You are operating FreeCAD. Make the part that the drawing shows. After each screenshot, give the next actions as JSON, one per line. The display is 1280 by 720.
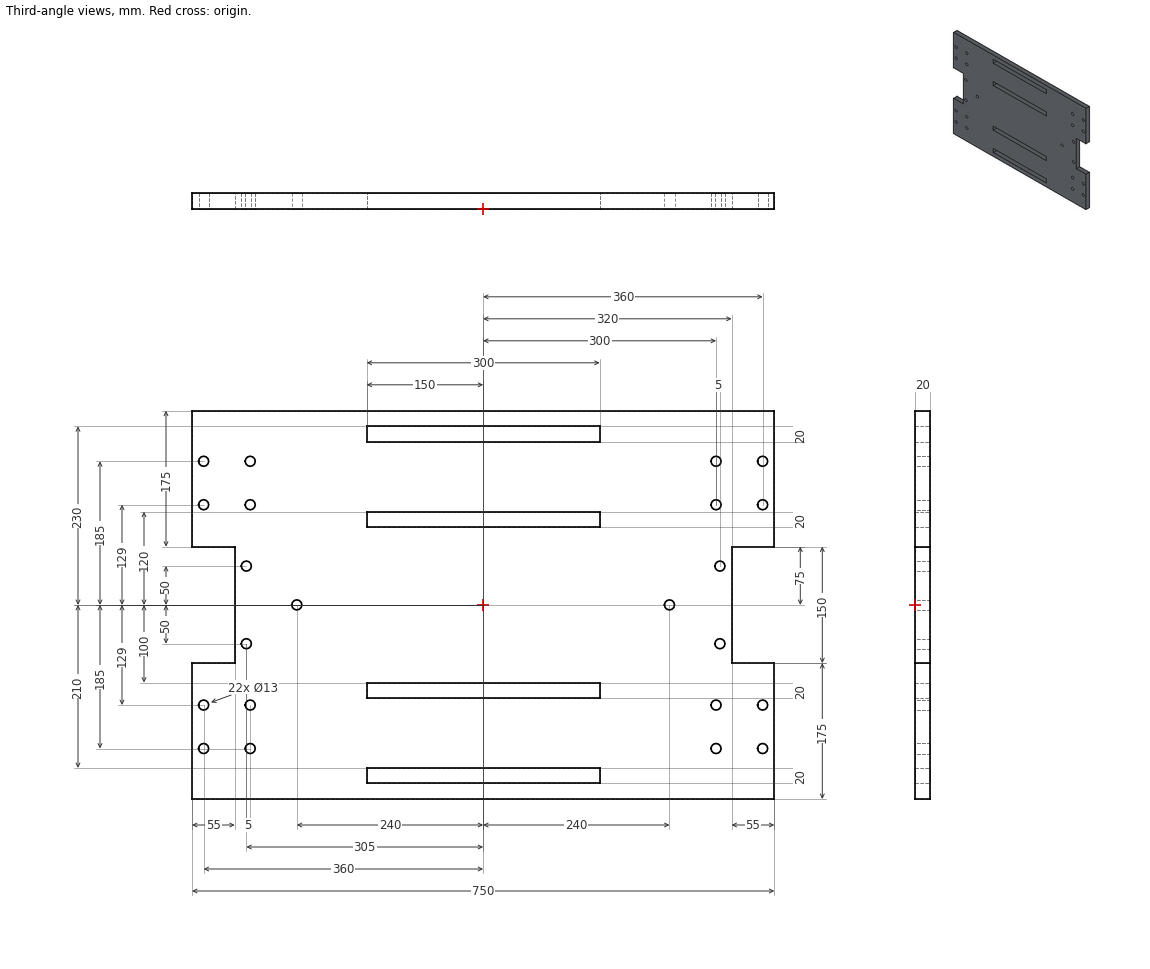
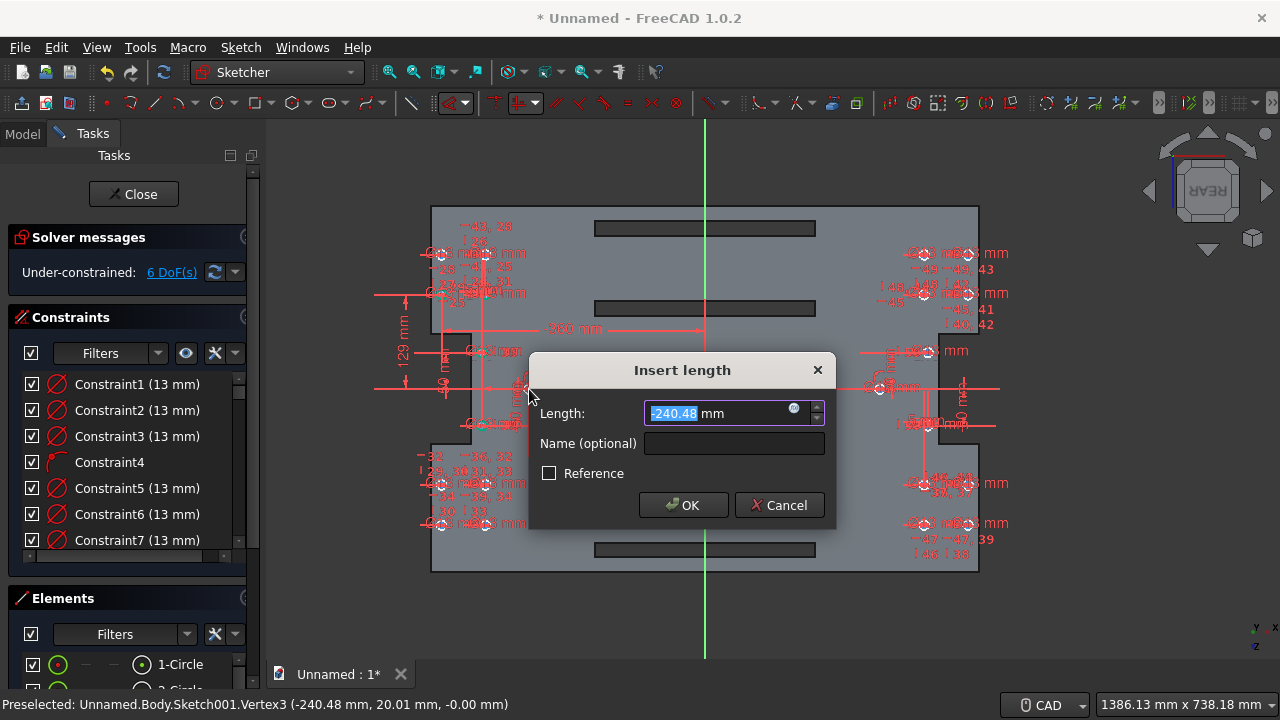
{"action": "type", "text": "-240"}
{"action": "key", "text": "Return"}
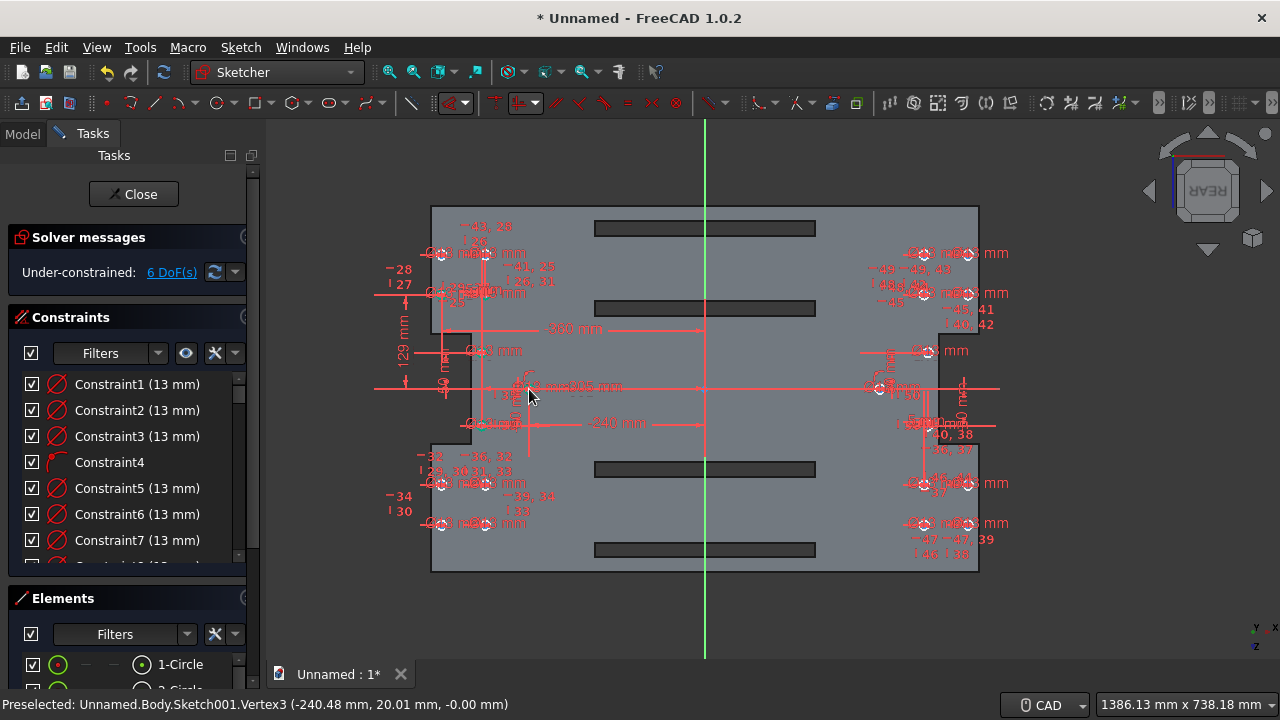
{"action": "left_click", "coordinate": [485, 255]}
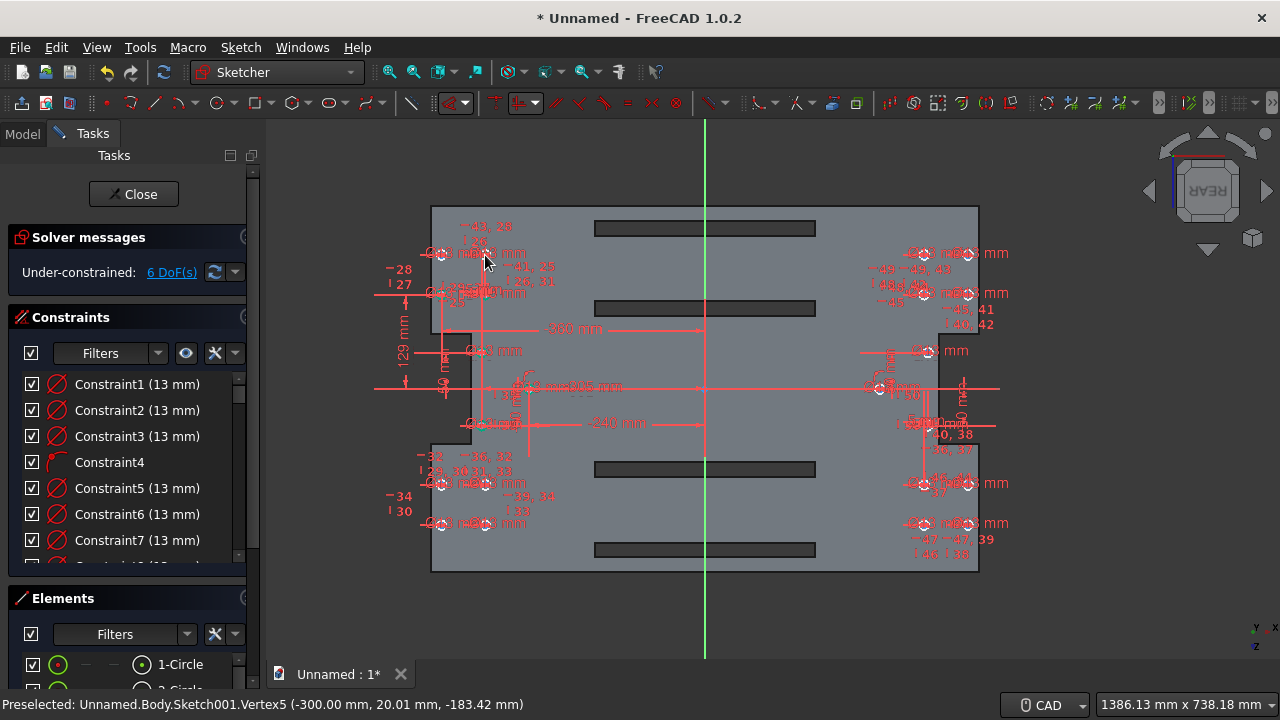
{"action": "left_click", "coordinate": [468, 104]}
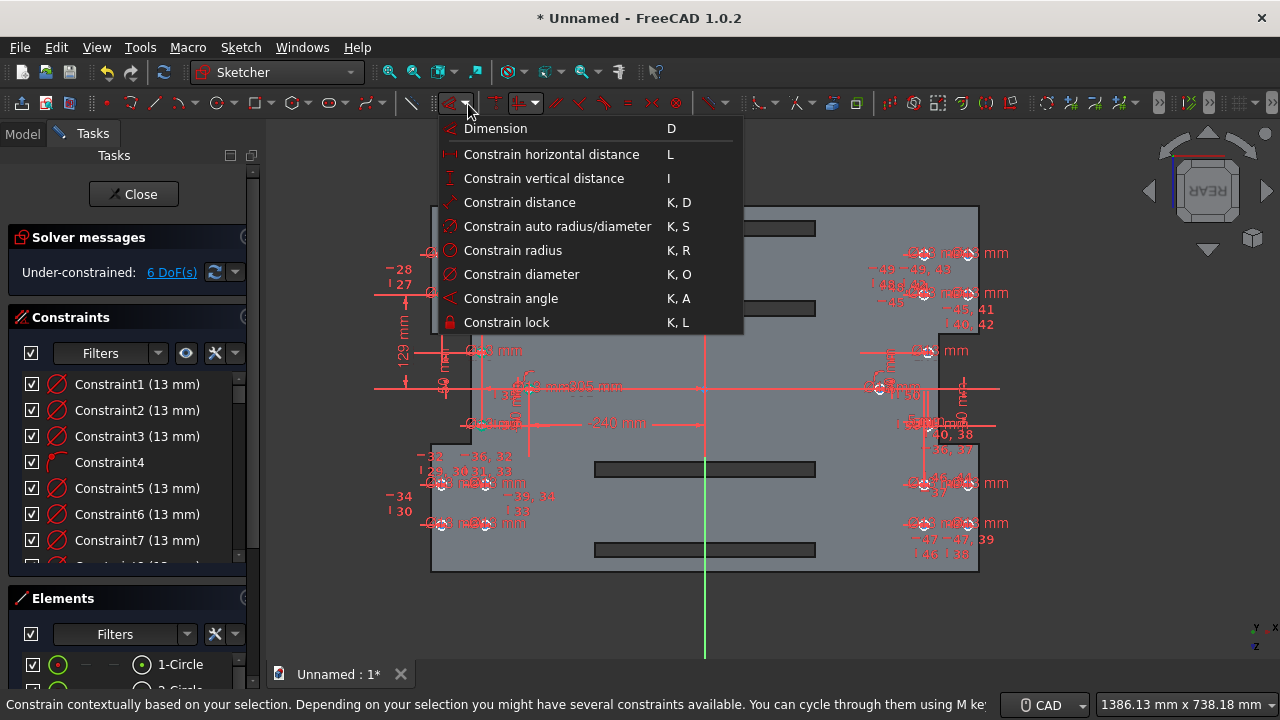
{"action": "left_click", "coordinate": [591, 178]}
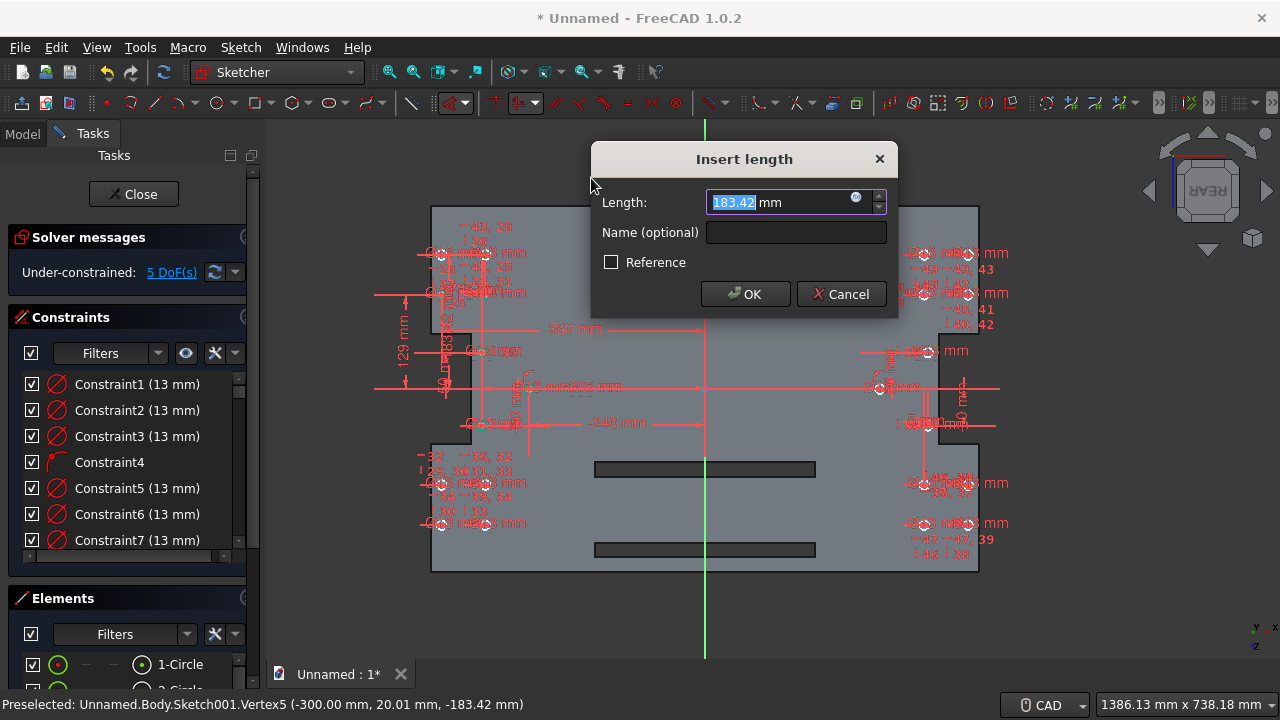
{"action": "type", "text": "185"}
{"action": "key", "text": "Return"}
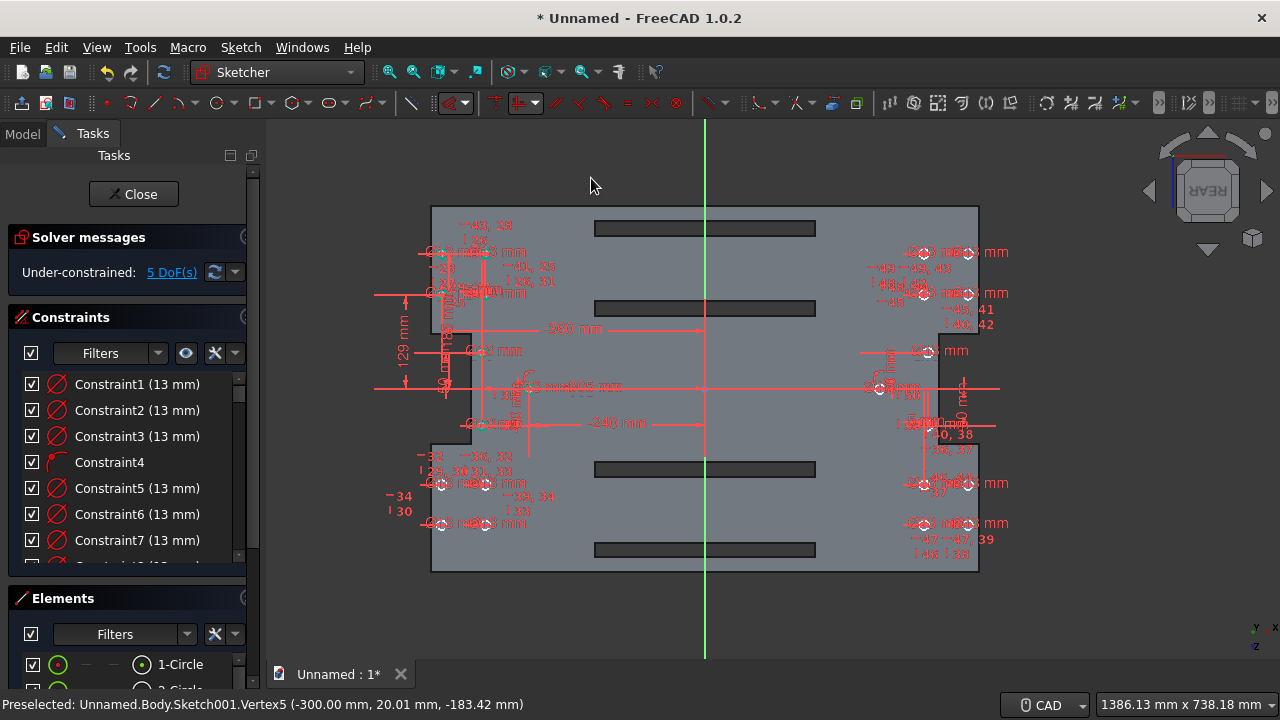
{"action": "left_click", "coordinate": [442, 485]}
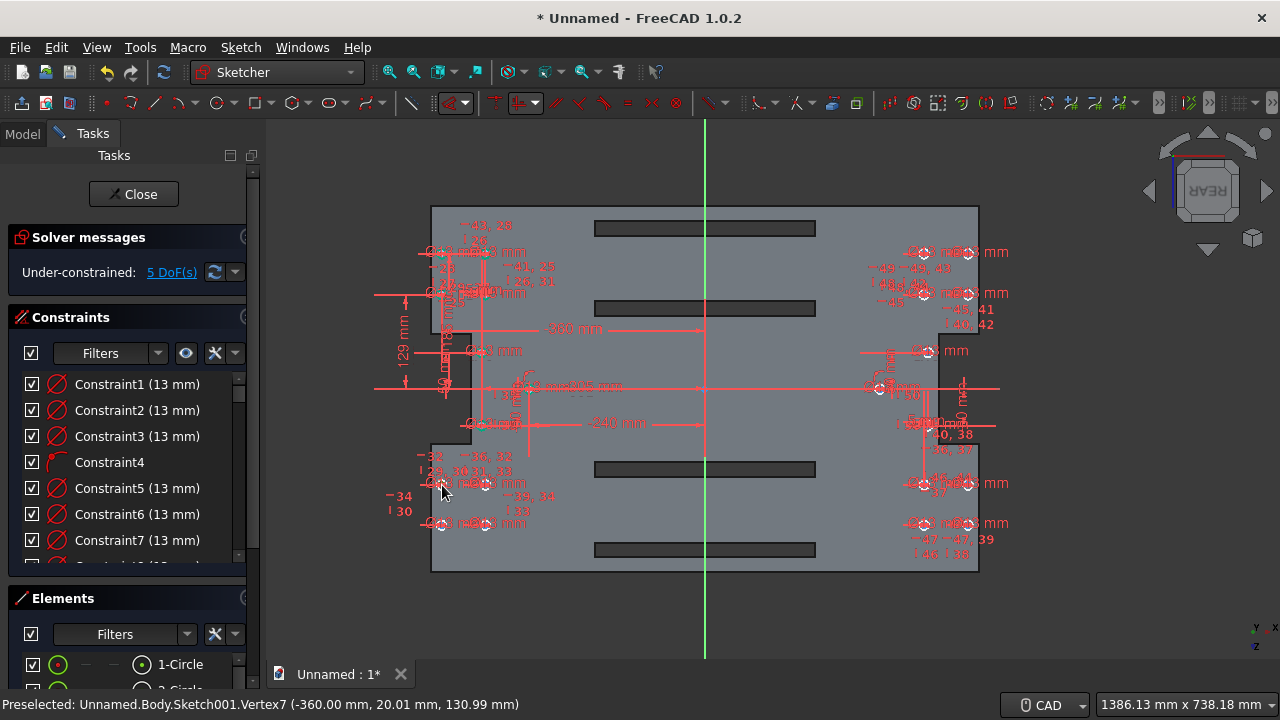
{"action": "left_click", "coordinate": [468, 104]}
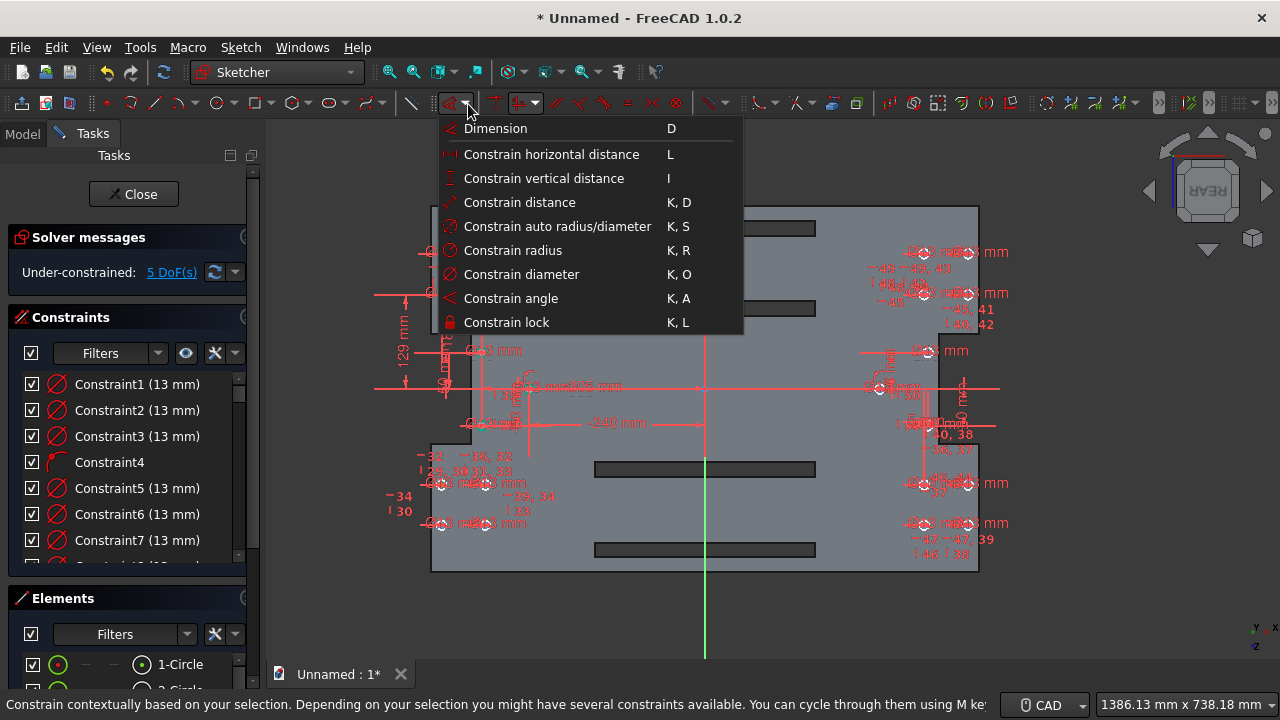
{"action": "left_click", "coordinate": [591, 178]}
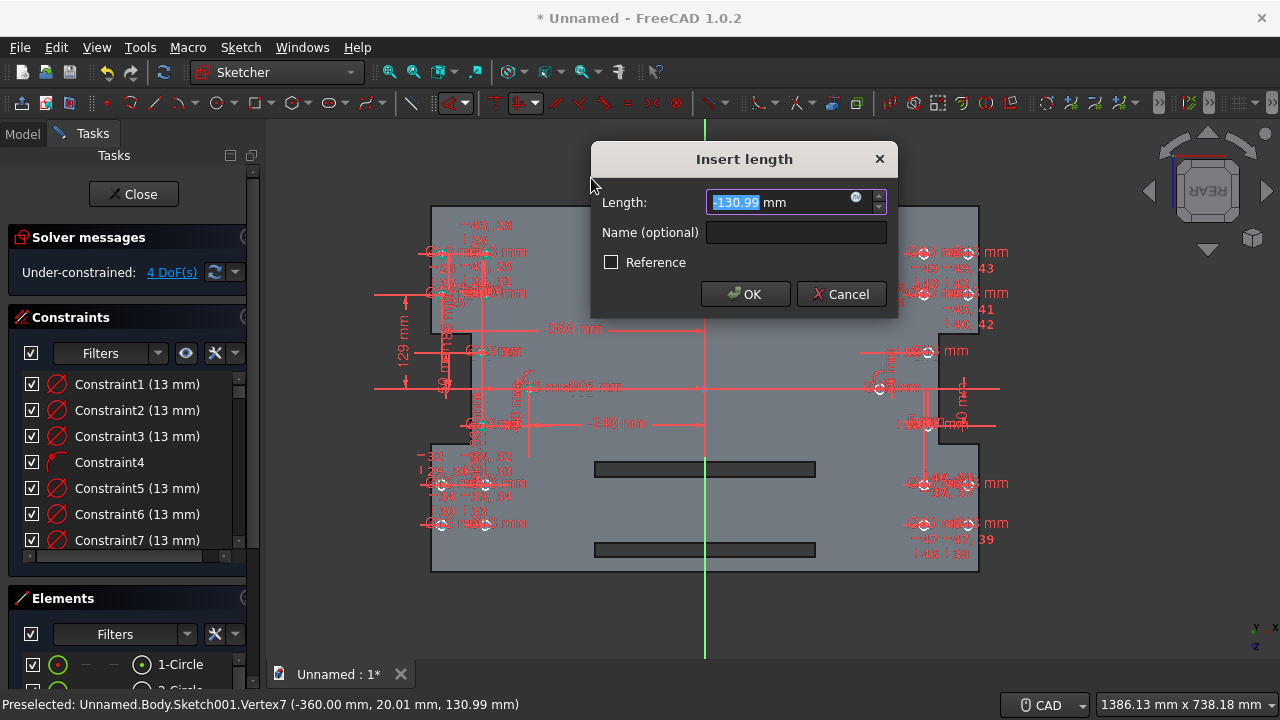
{"action": "type", "text": "-129"}
{"action": "key", "text": "Return"}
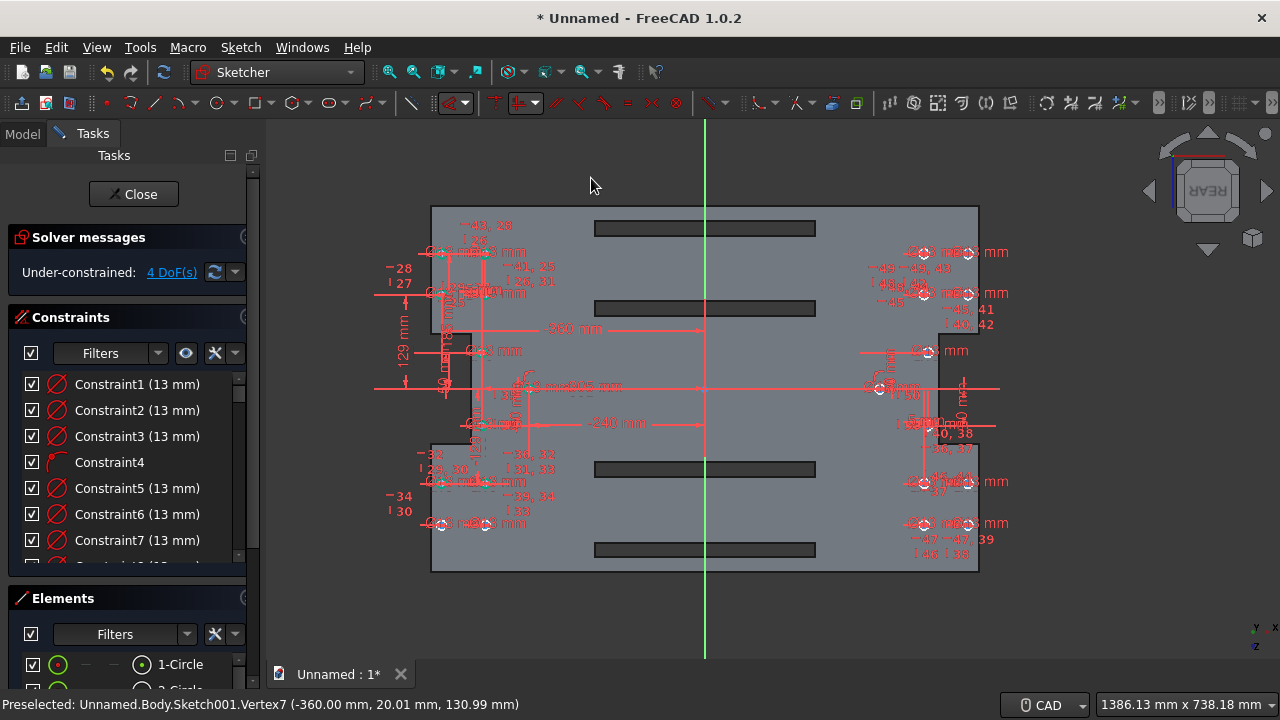
{"action": "left_click", "coordinate": [442, 525]}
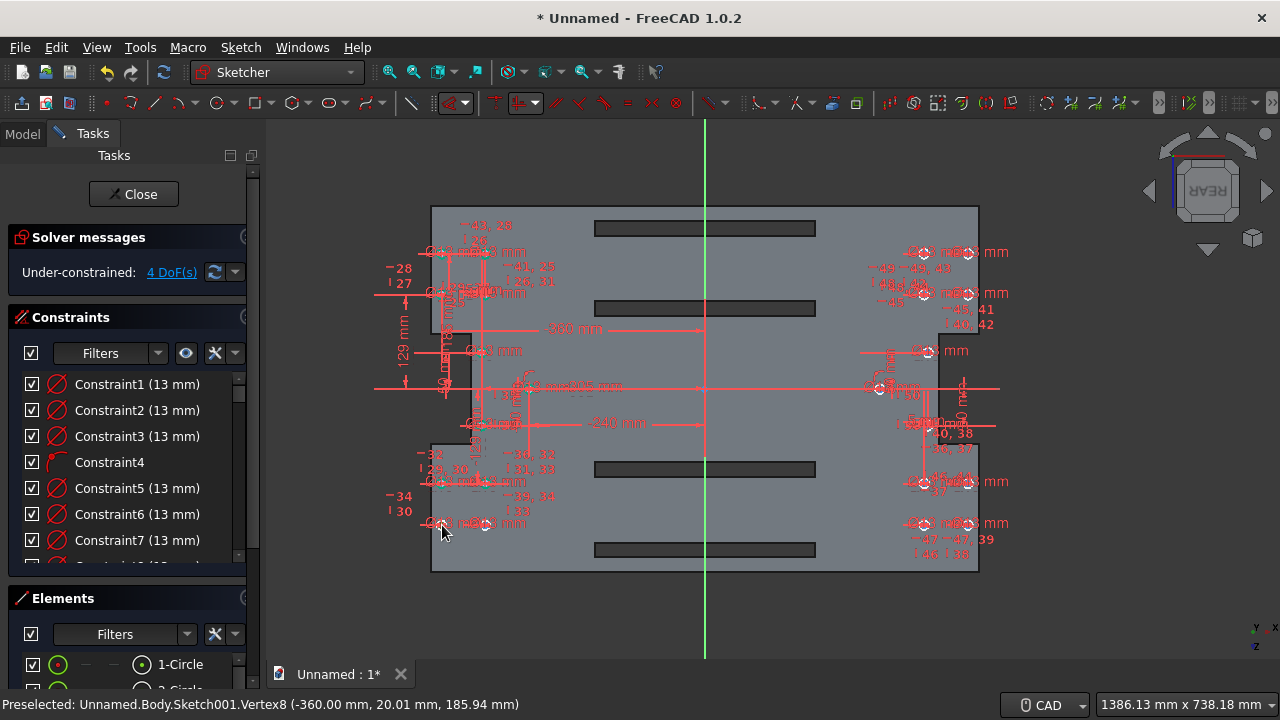
{"action": "left_click", "coordinate": [468, 104]}